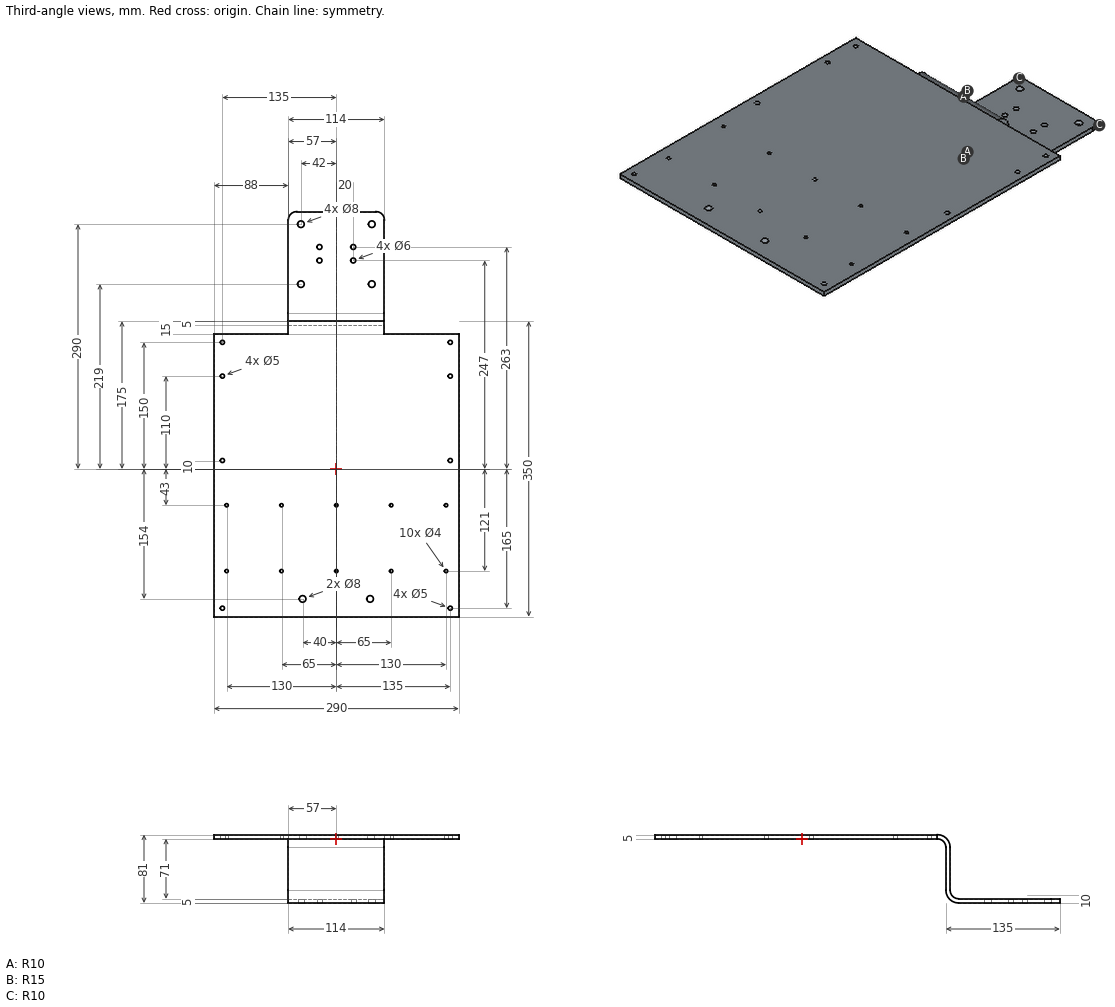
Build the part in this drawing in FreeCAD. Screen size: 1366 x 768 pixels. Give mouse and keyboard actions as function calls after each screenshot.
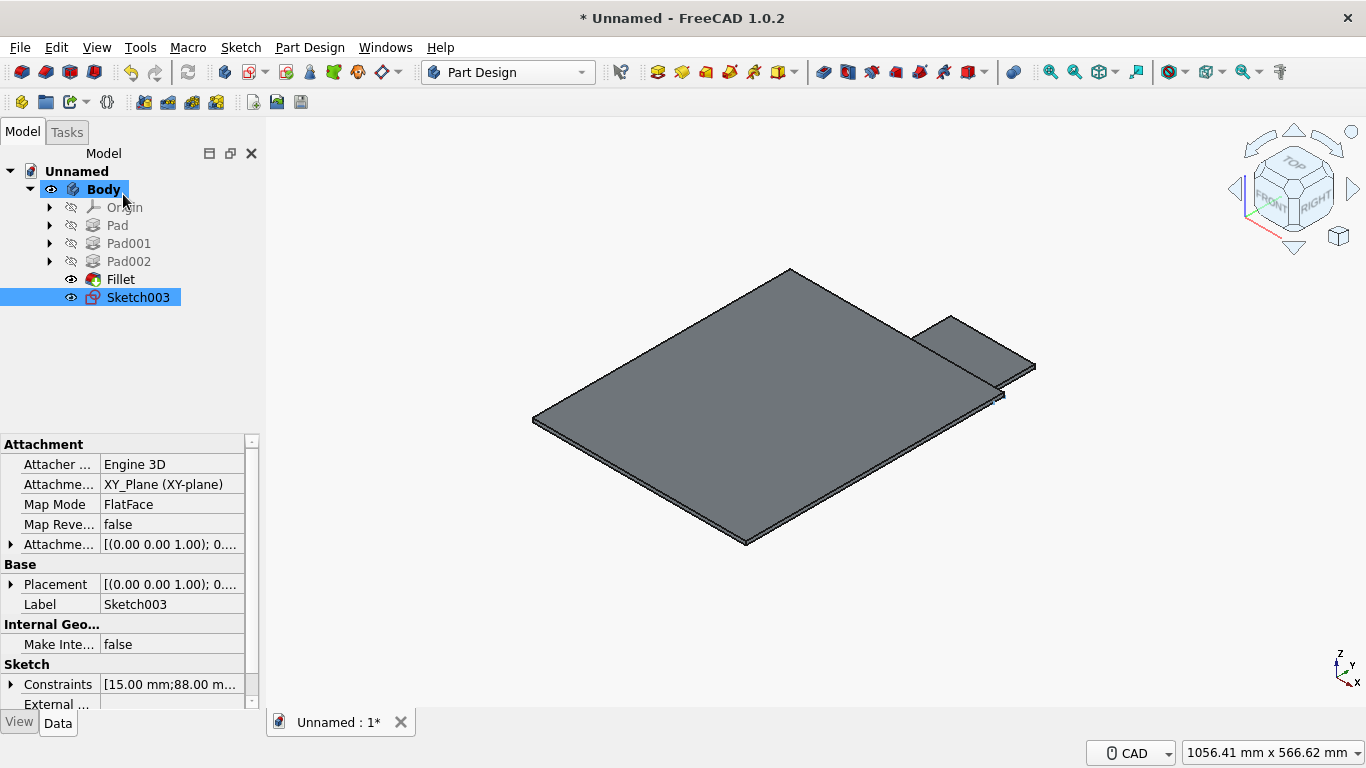
click(824, 72)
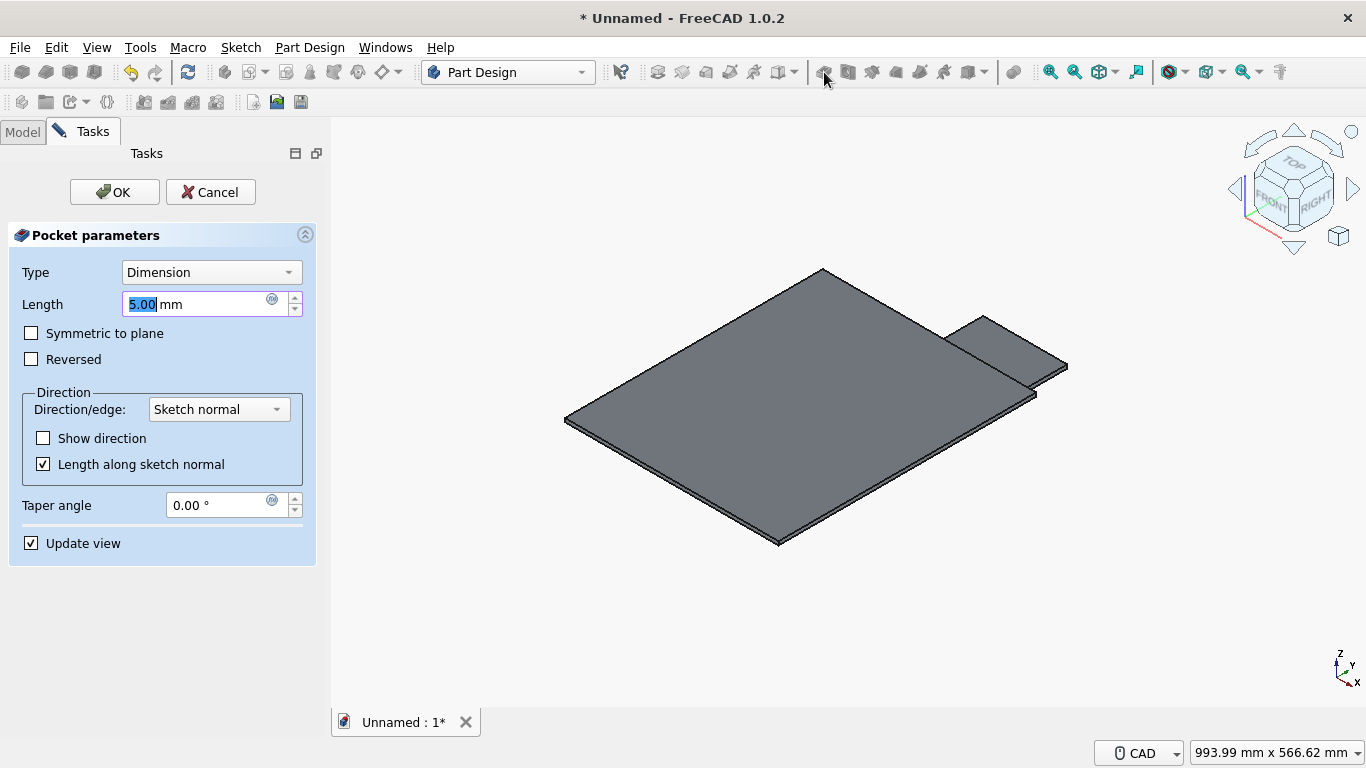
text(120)
key(Tab)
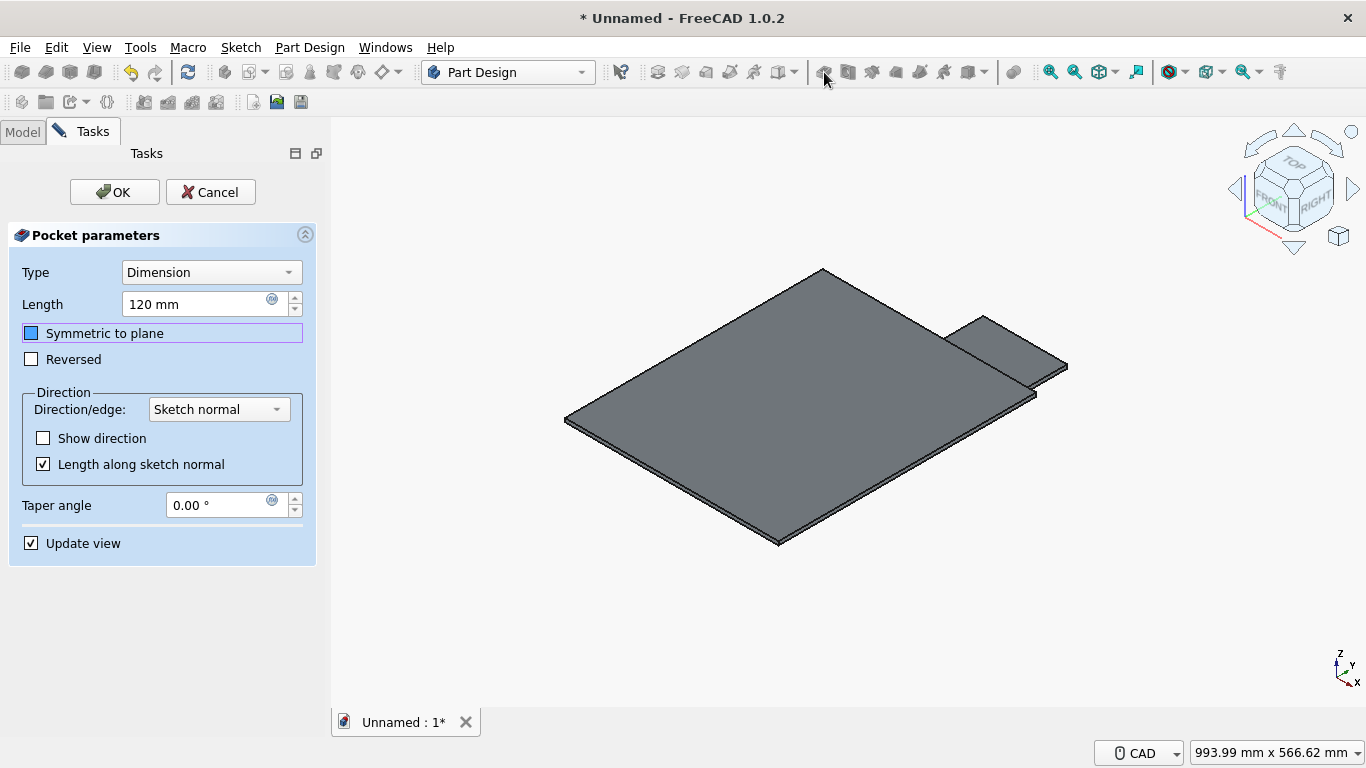
click(30, 359)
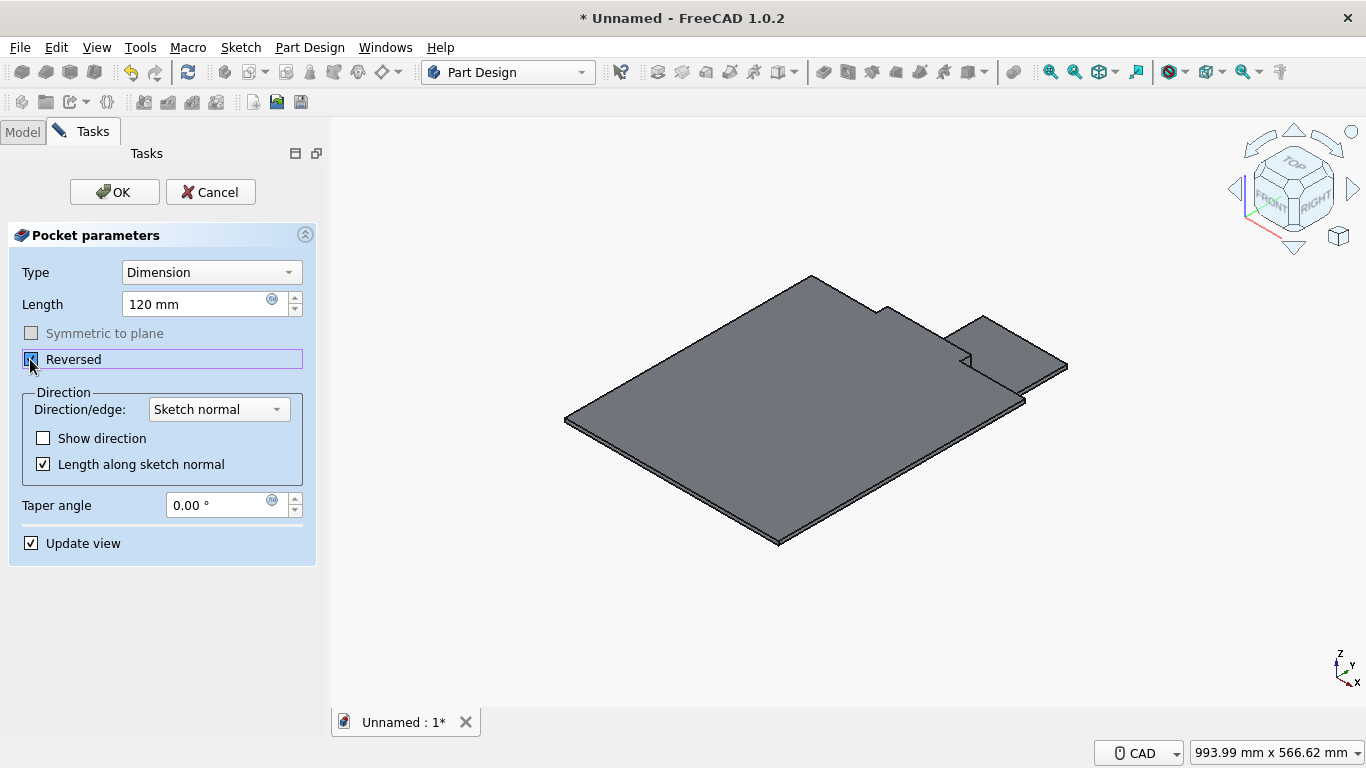
click(115, 192)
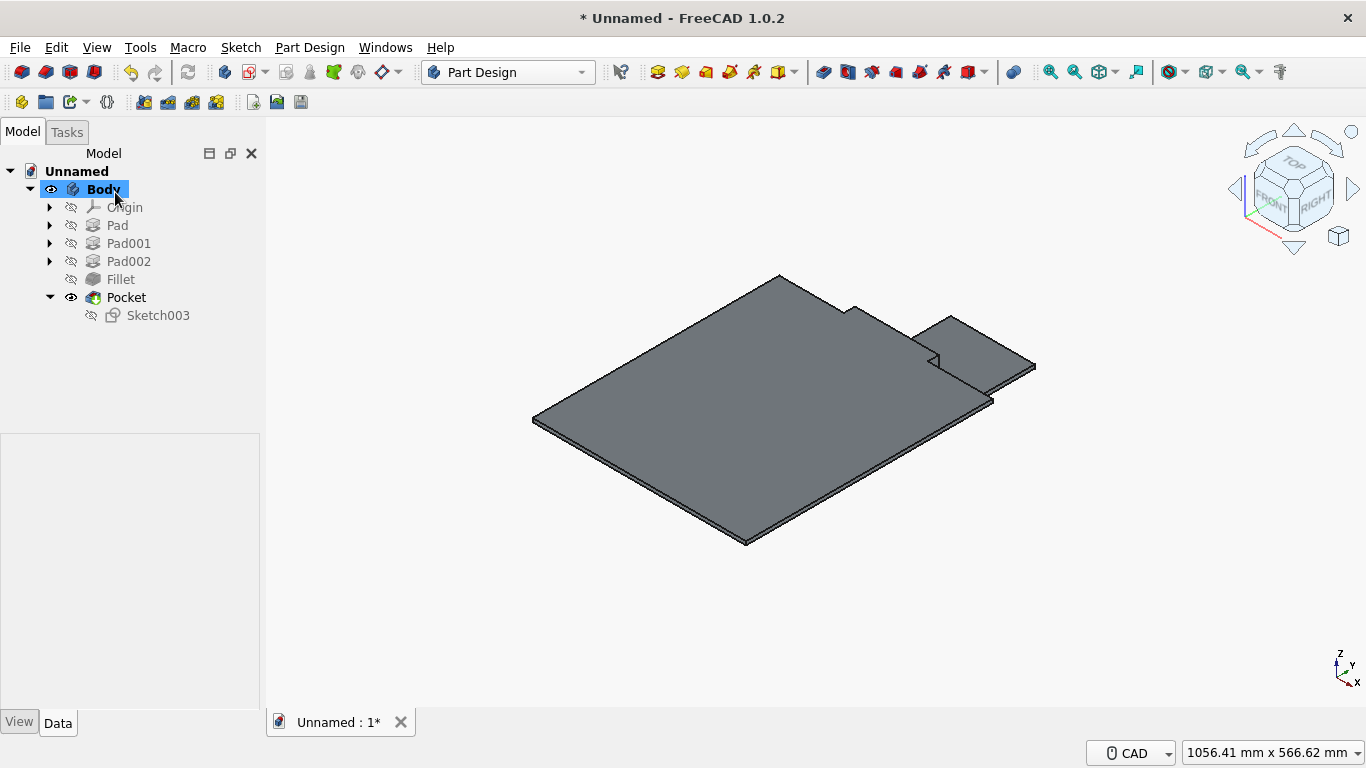
key(2)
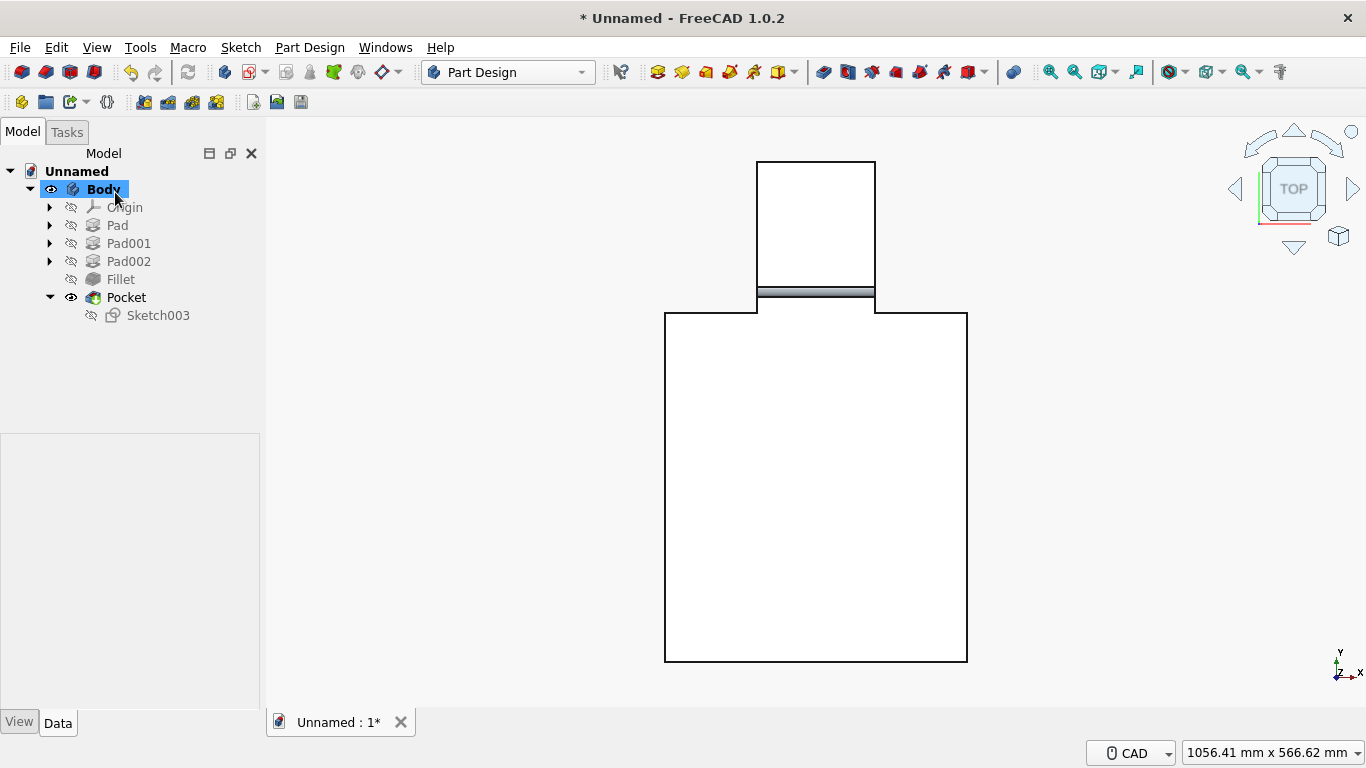
click(816, 296)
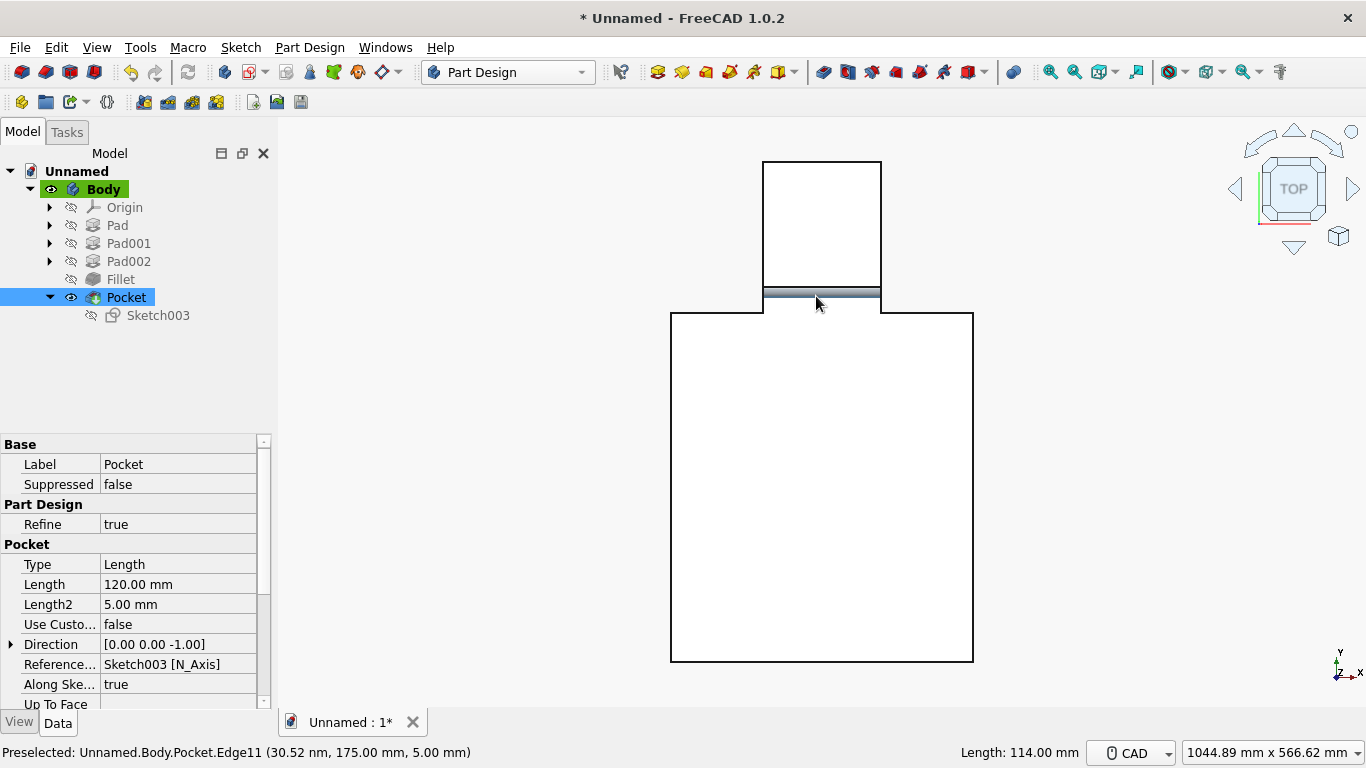
key(0)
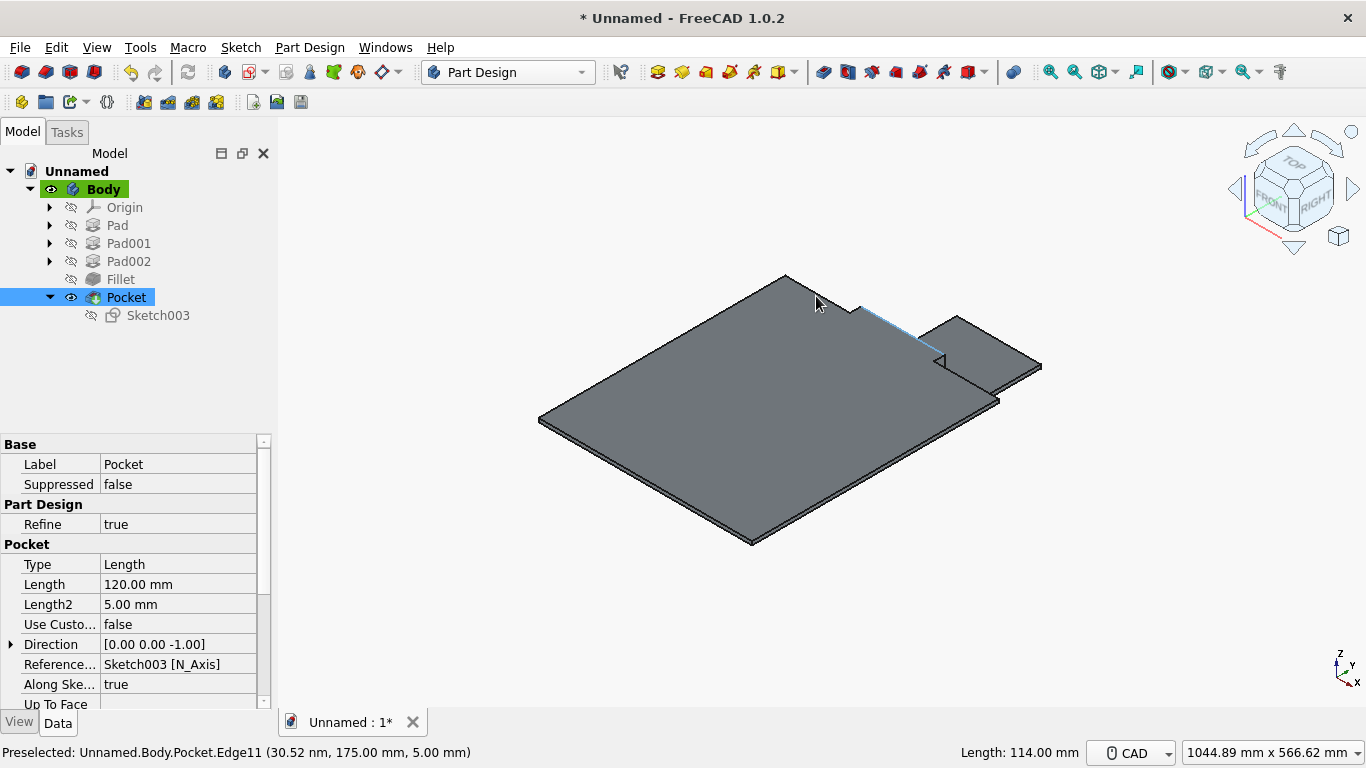
key(1)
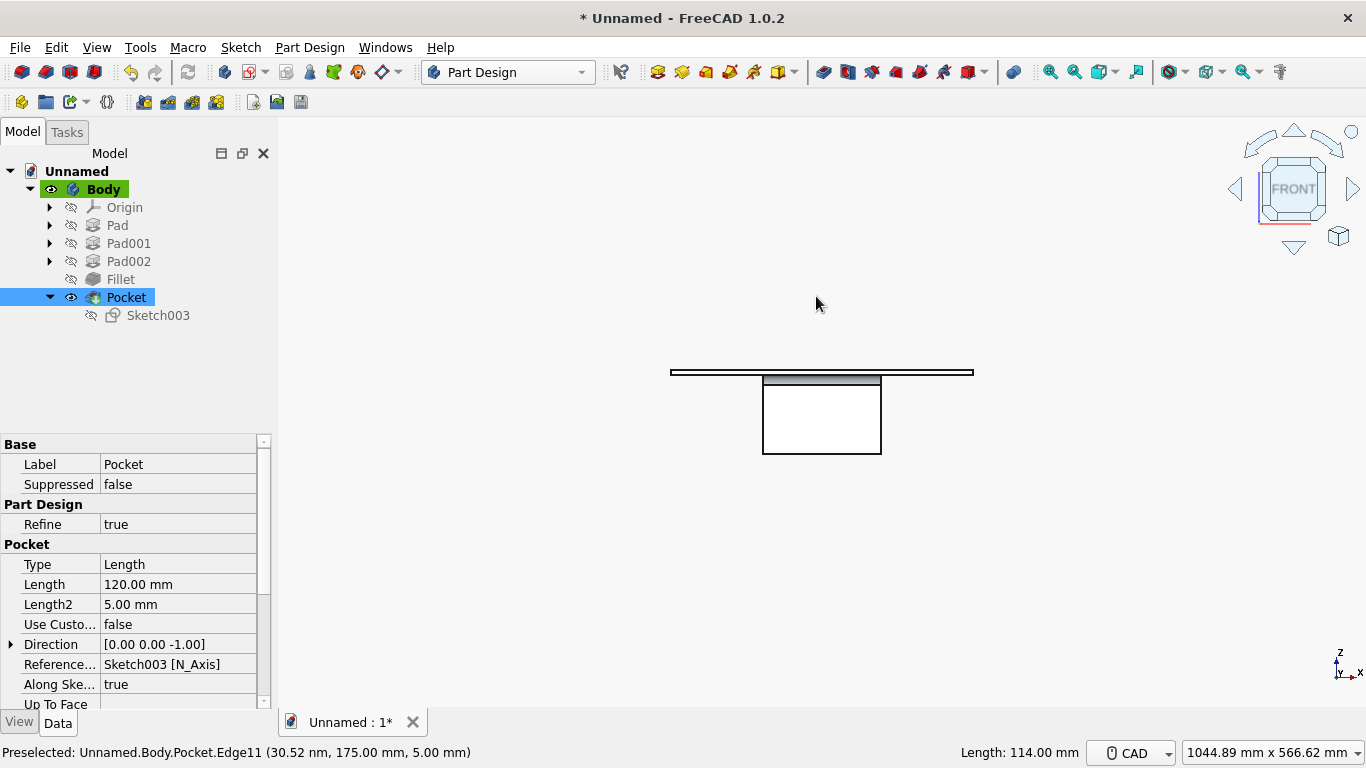
click(1052, 72)